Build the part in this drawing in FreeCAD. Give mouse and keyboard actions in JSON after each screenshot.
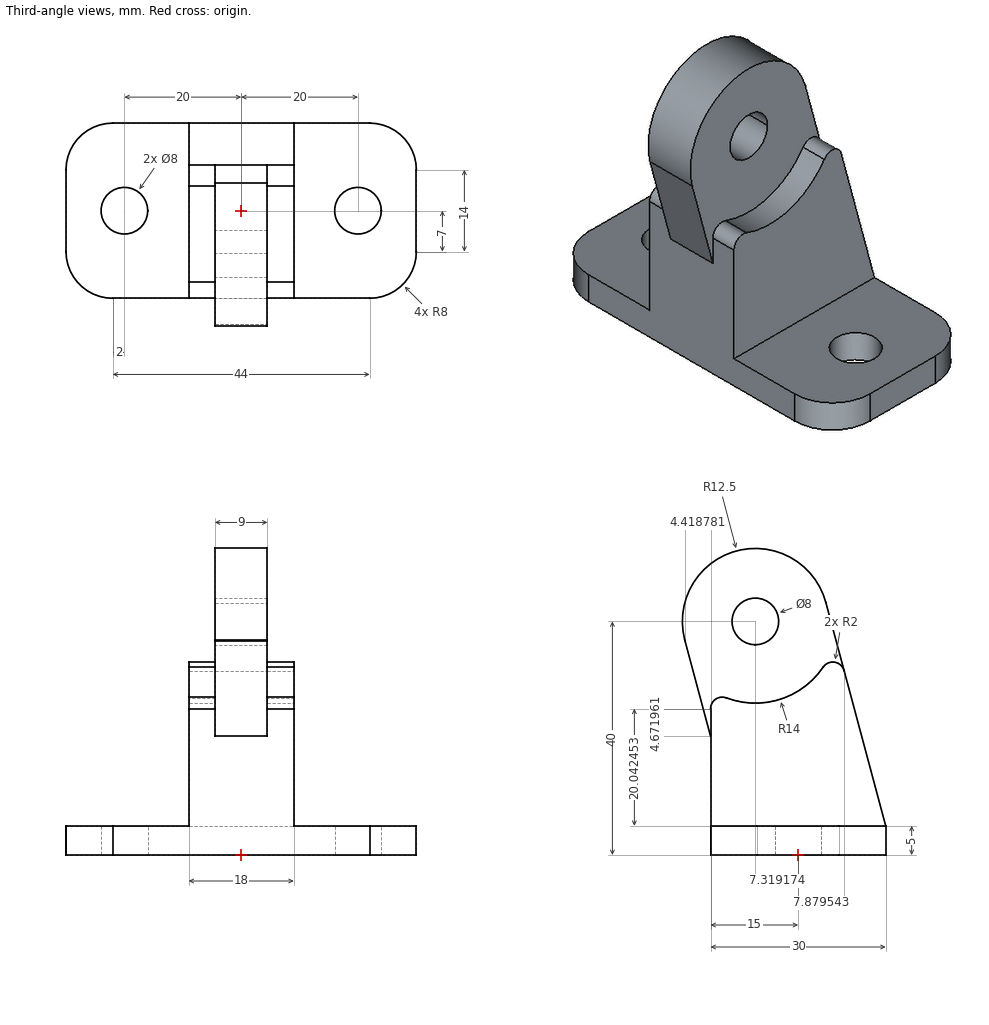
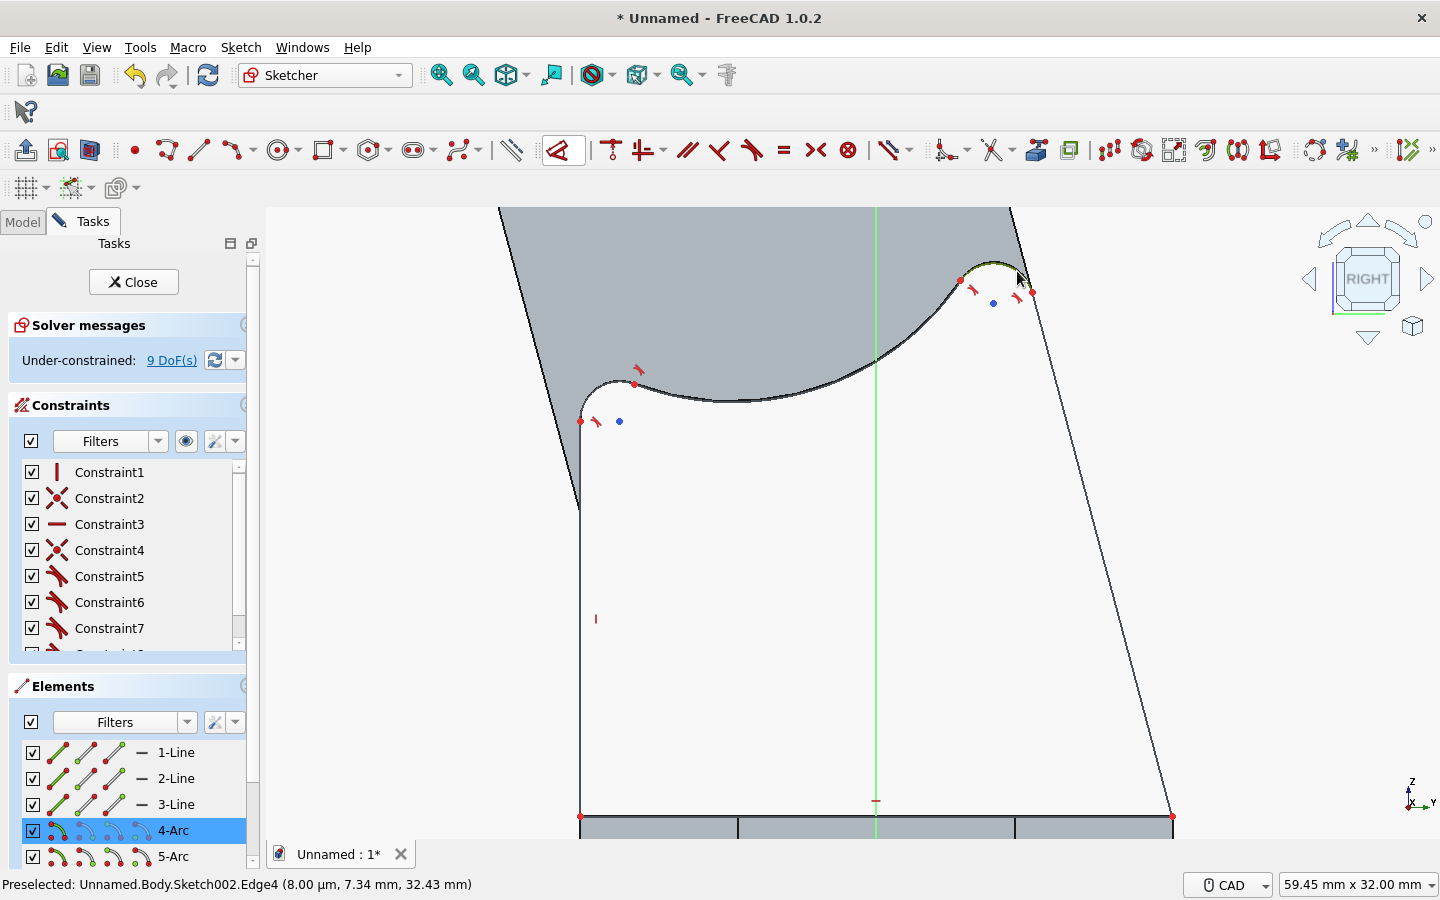
{"action": "left_click", "coordinate": [611, 382]}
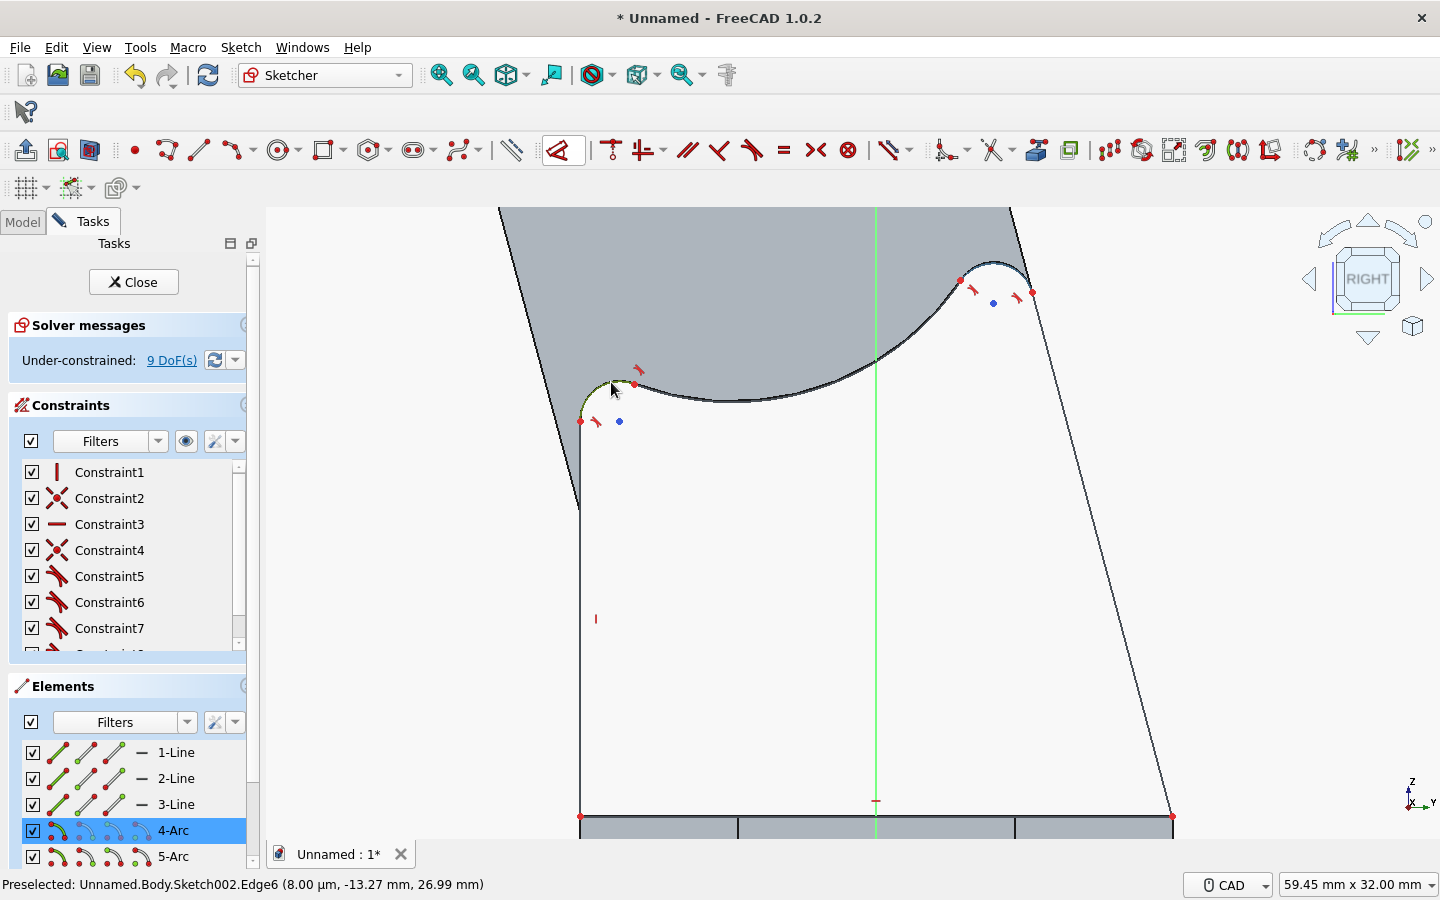
{"action": "key", "text": "e"}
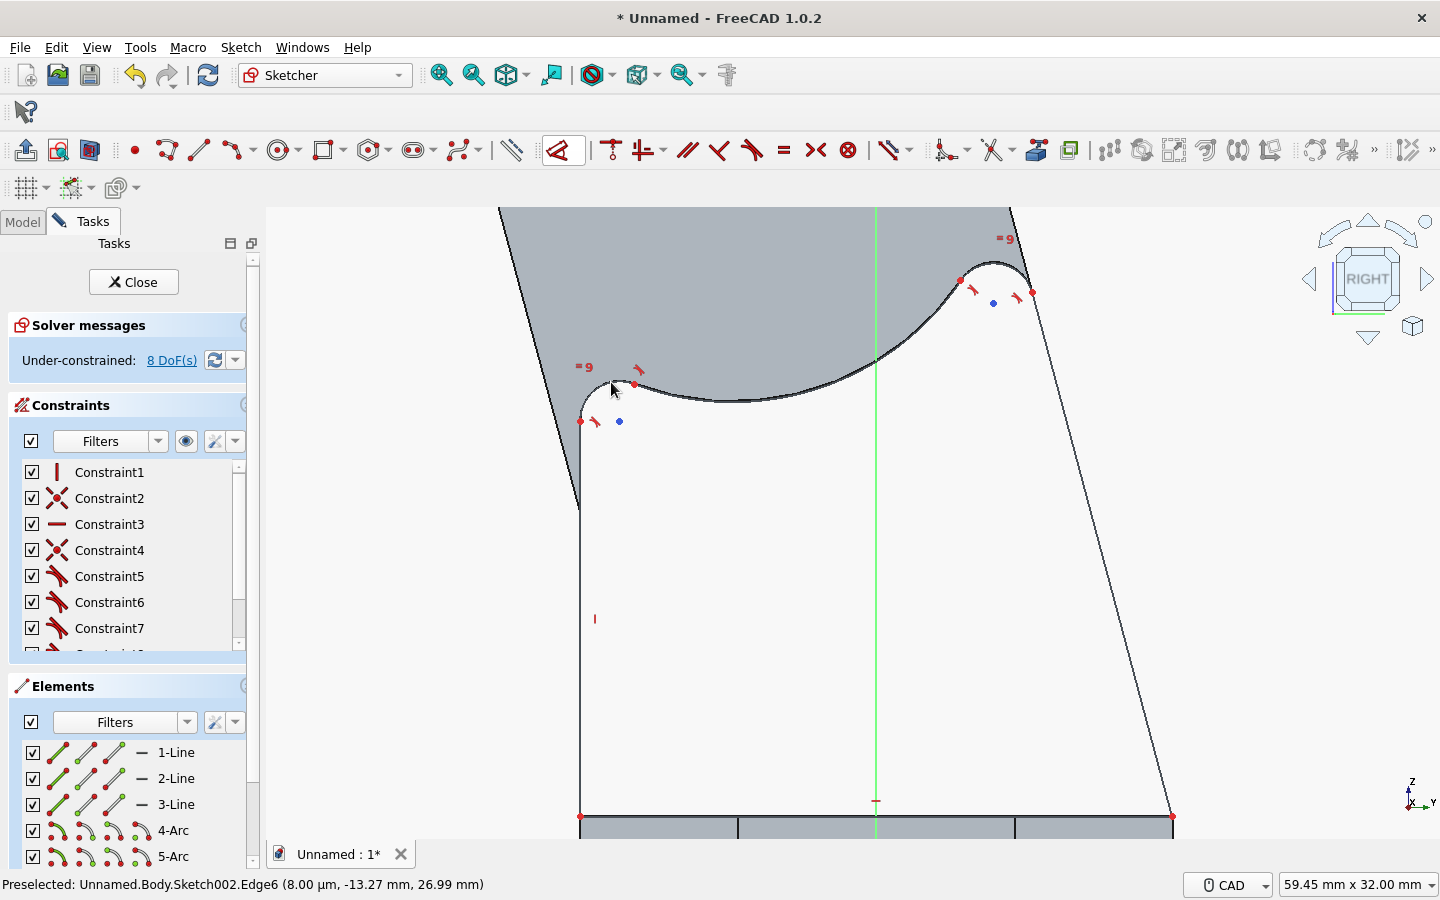
{"action": "left_click", "coordinate": [1017, 271]}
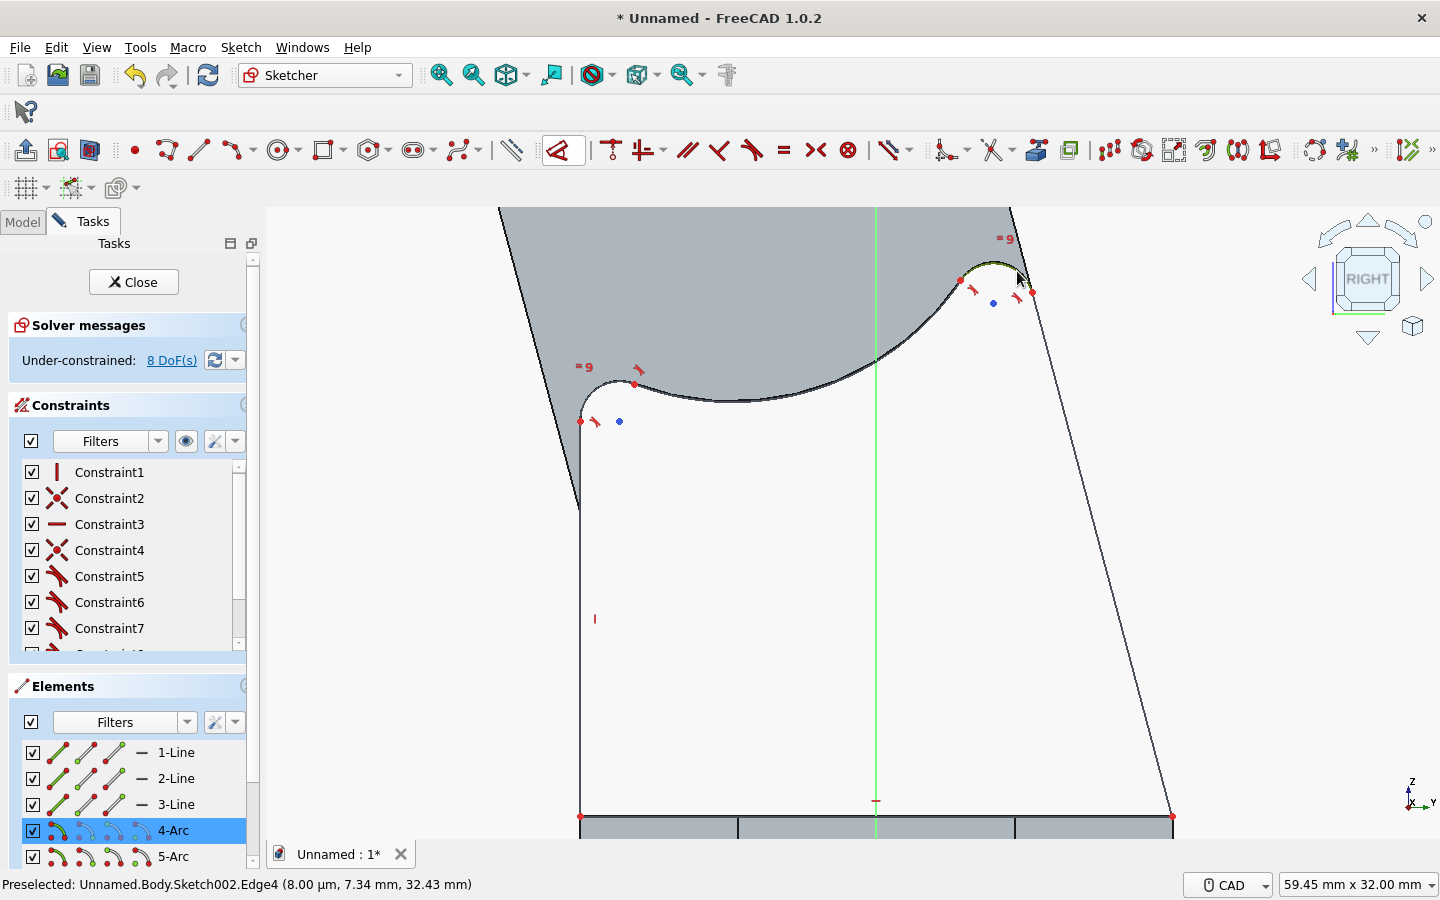
{"action": "key", "text": "k r"}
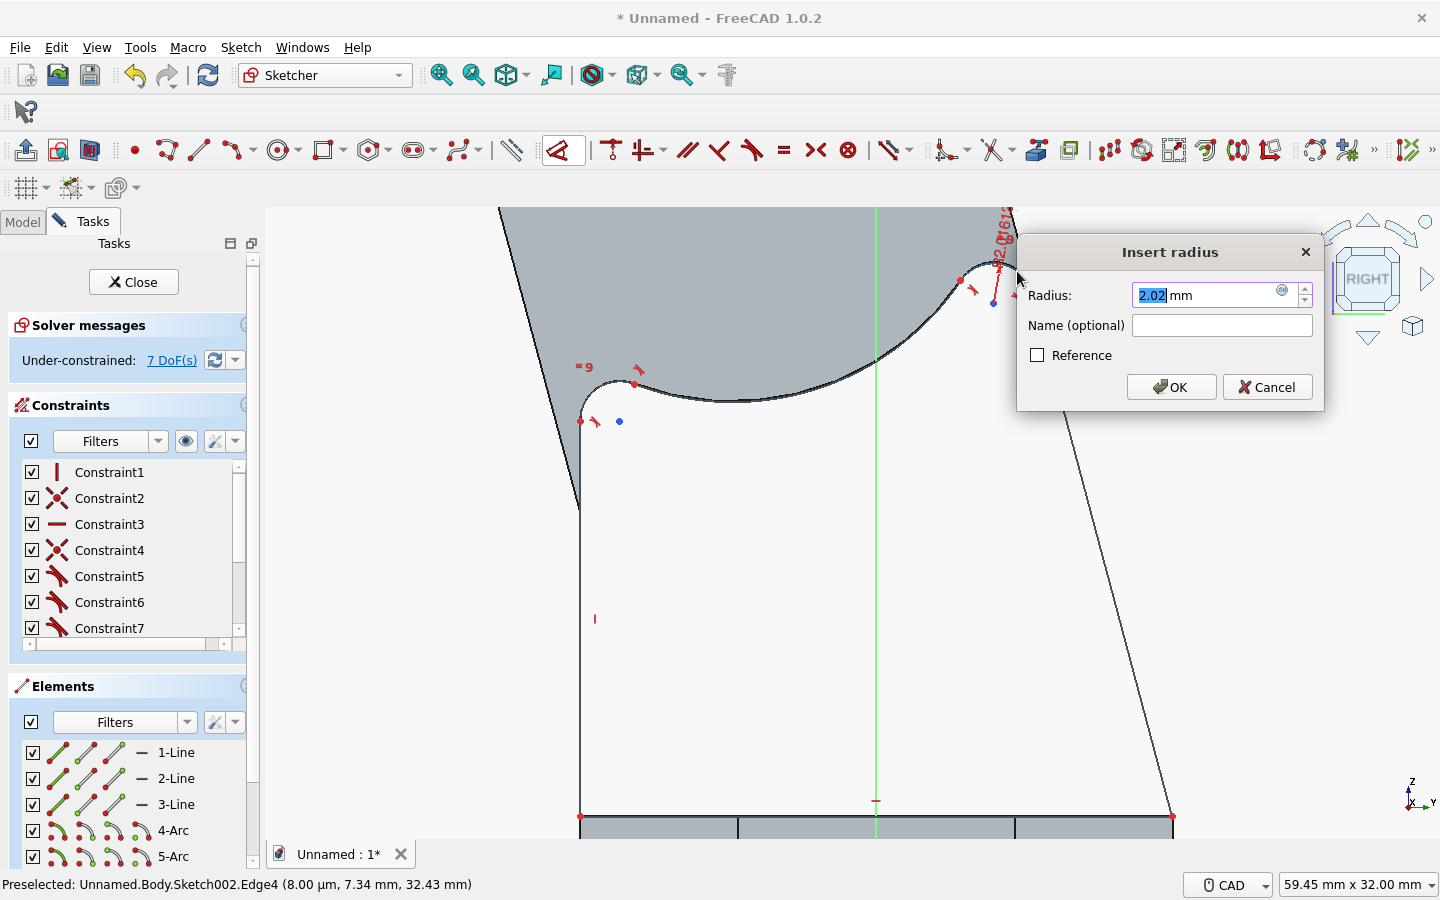
{"action": "type", "text": "2"}
{"action": "key", "text": "Return"}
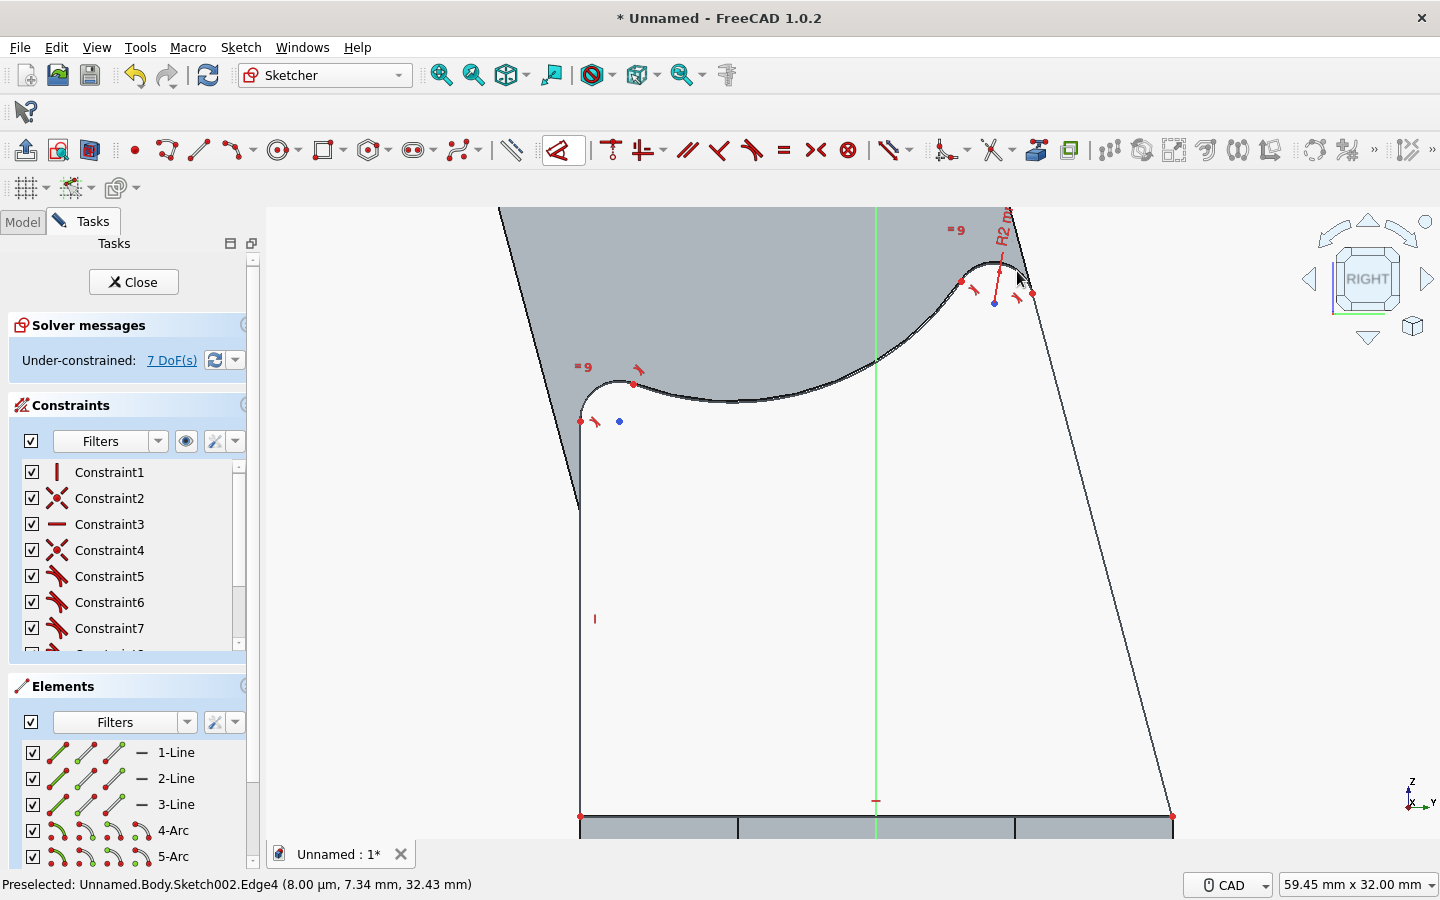
{"action": "left_click", "coordinate": [743, 402]}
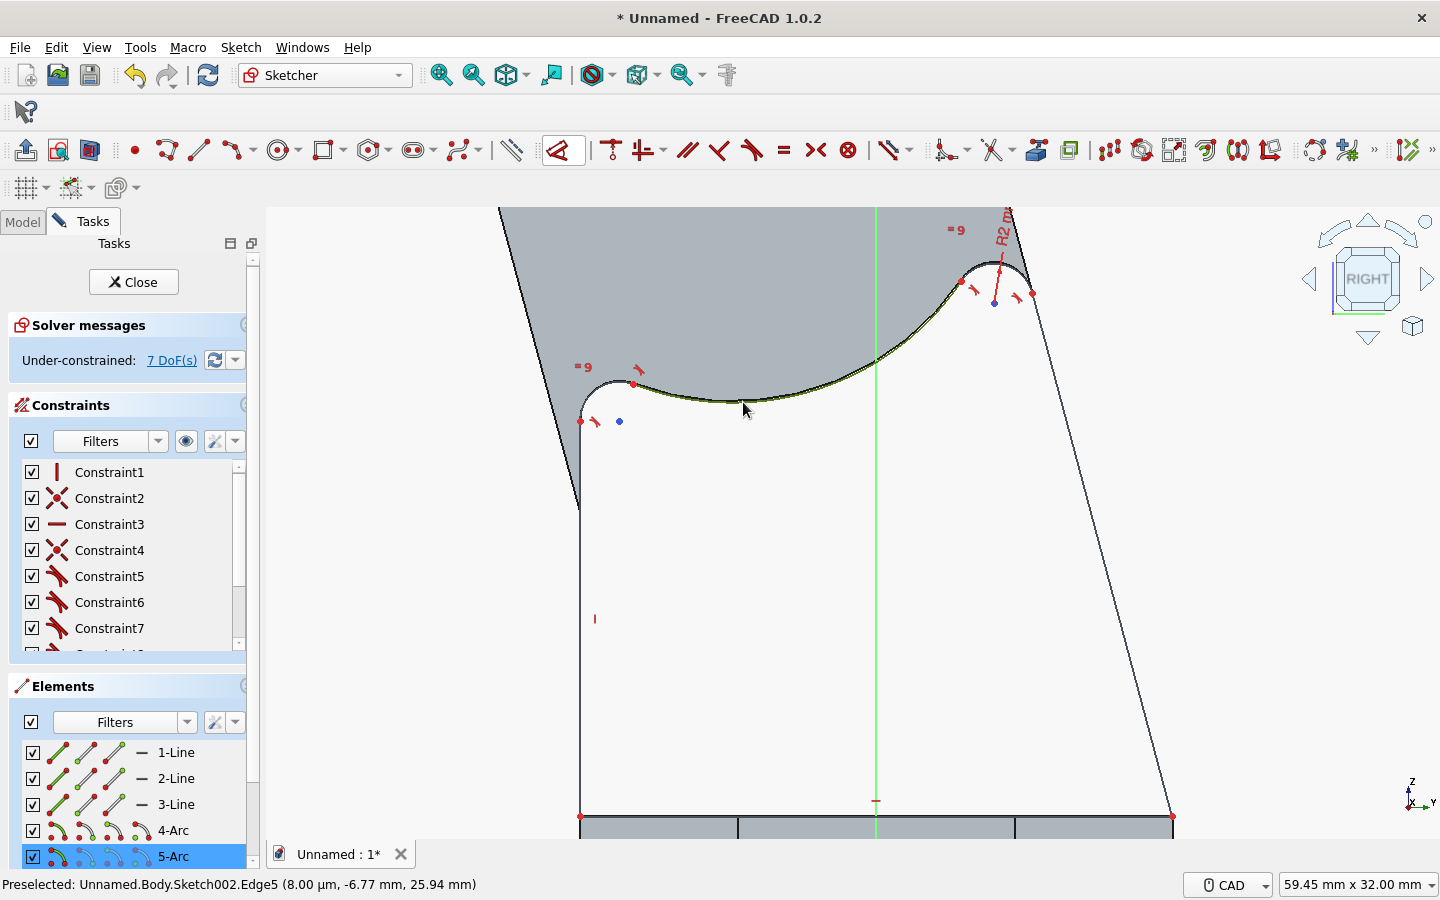
{"action": "key", "text": "k r"}